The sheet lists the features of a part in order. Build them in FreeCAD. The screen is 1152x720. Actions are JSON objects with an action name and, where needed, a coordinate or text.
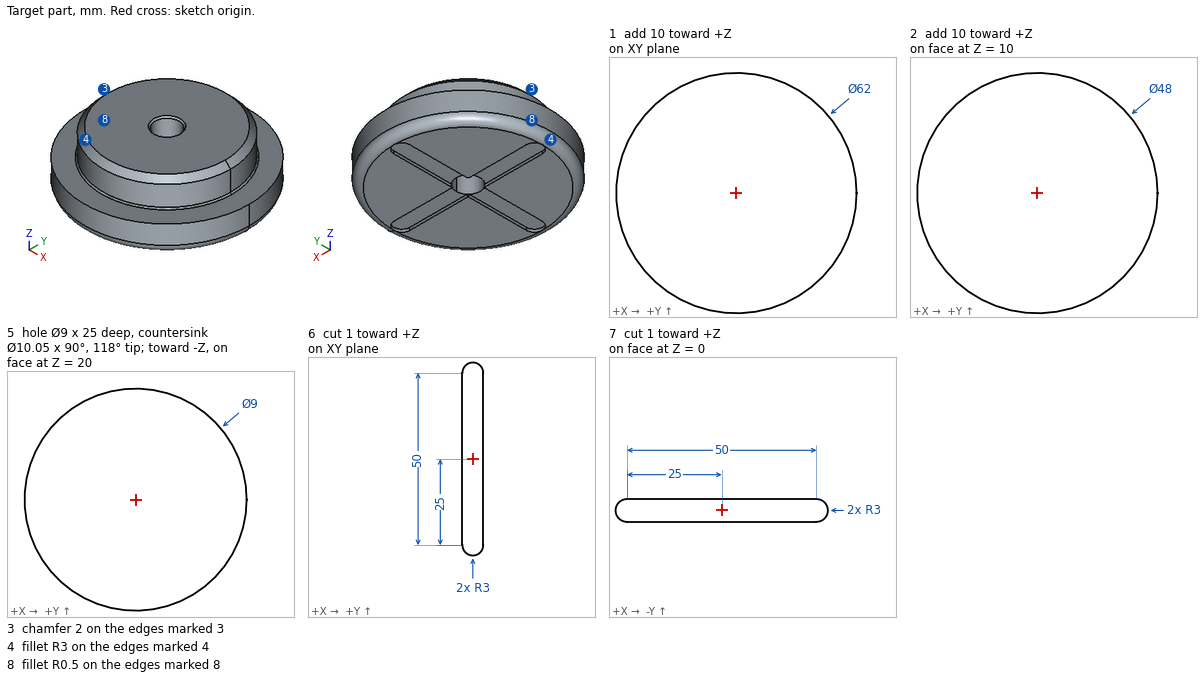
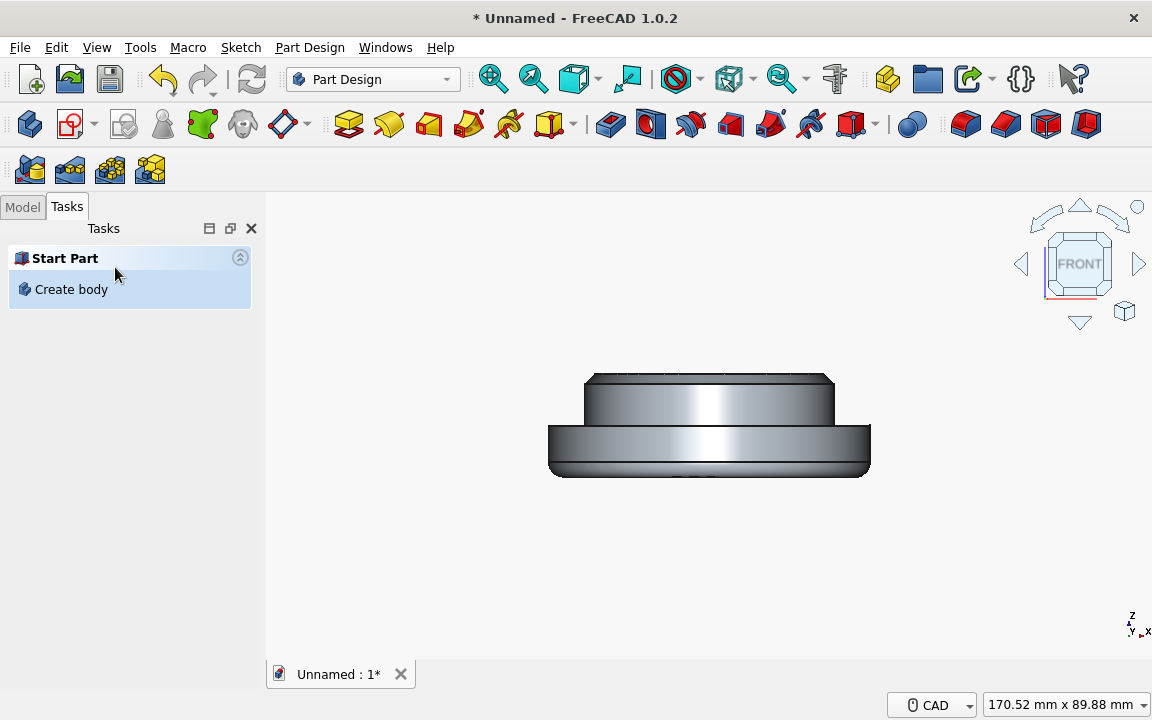
{"action": "left_click", "coordinate": [494, 80]}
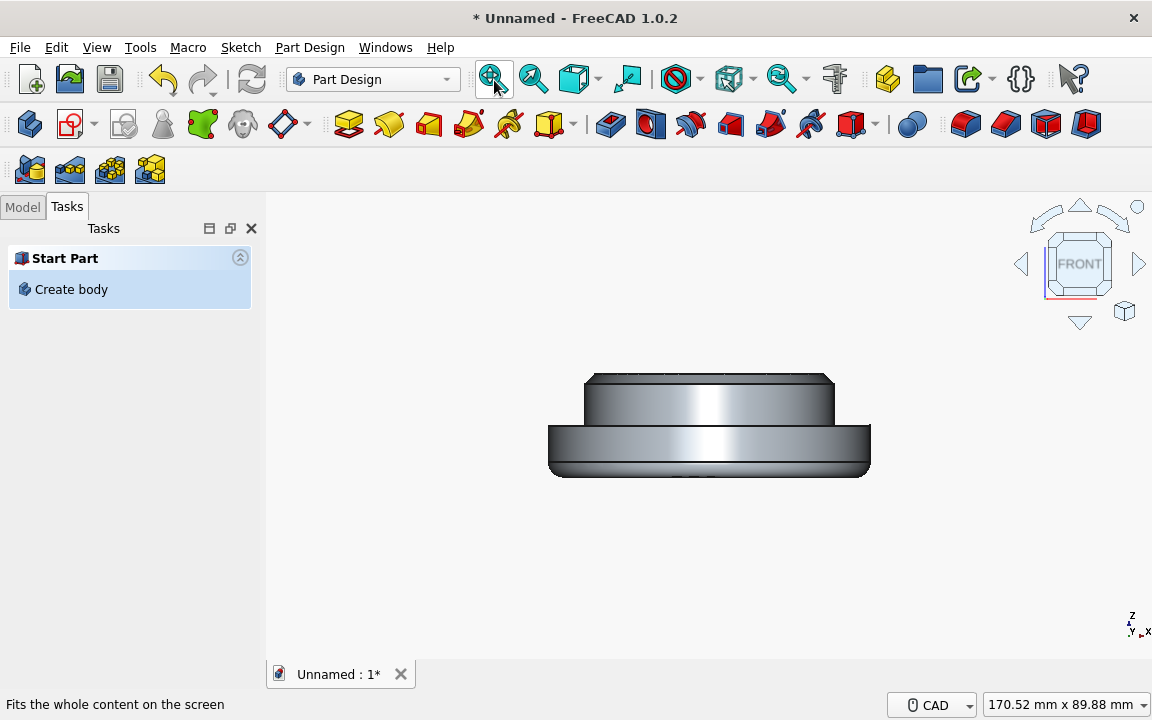
{"action": "key", "text": "3"}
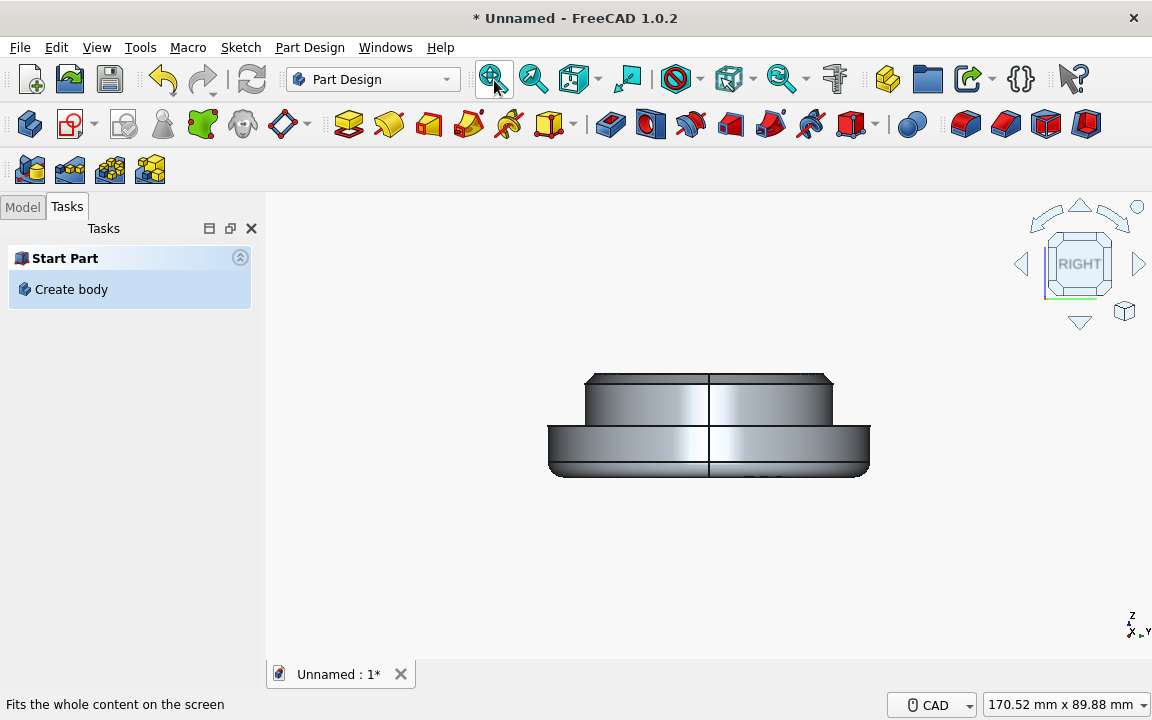
{"action": "left_click", "coordinate": [494, 80]}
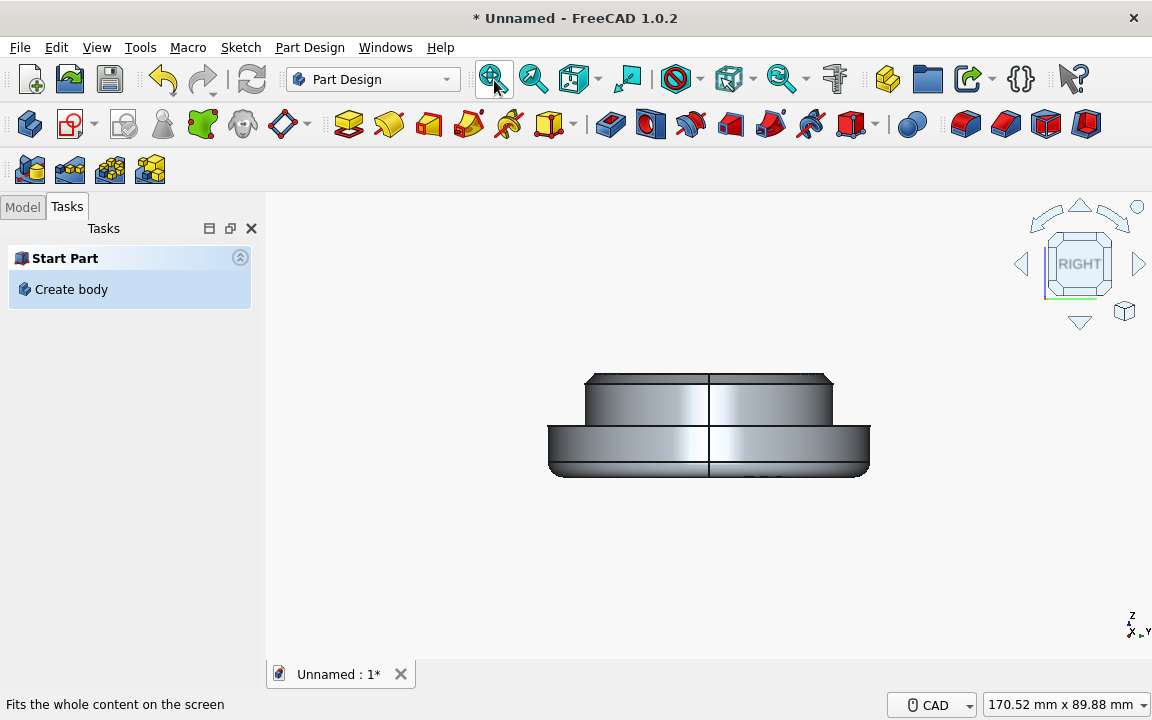
{"action": "key", "text": "5"}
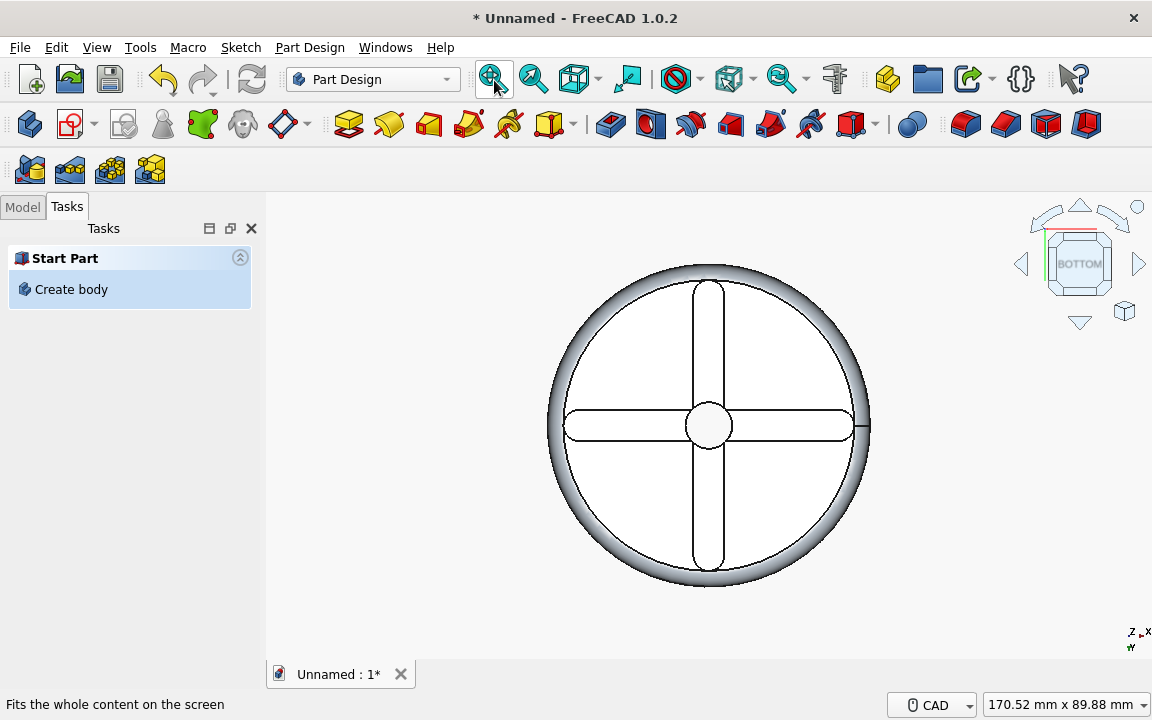
{"action": "key", "text": "4"}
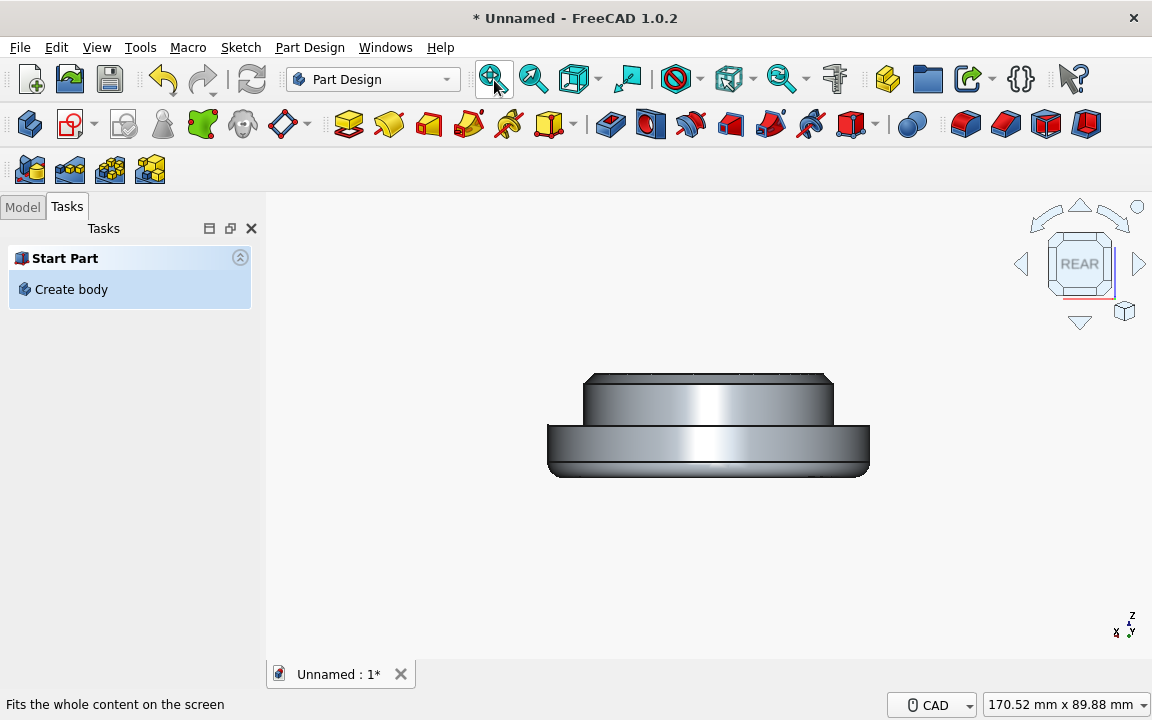
{"action": "left_click", "coordinate": [494, 80]}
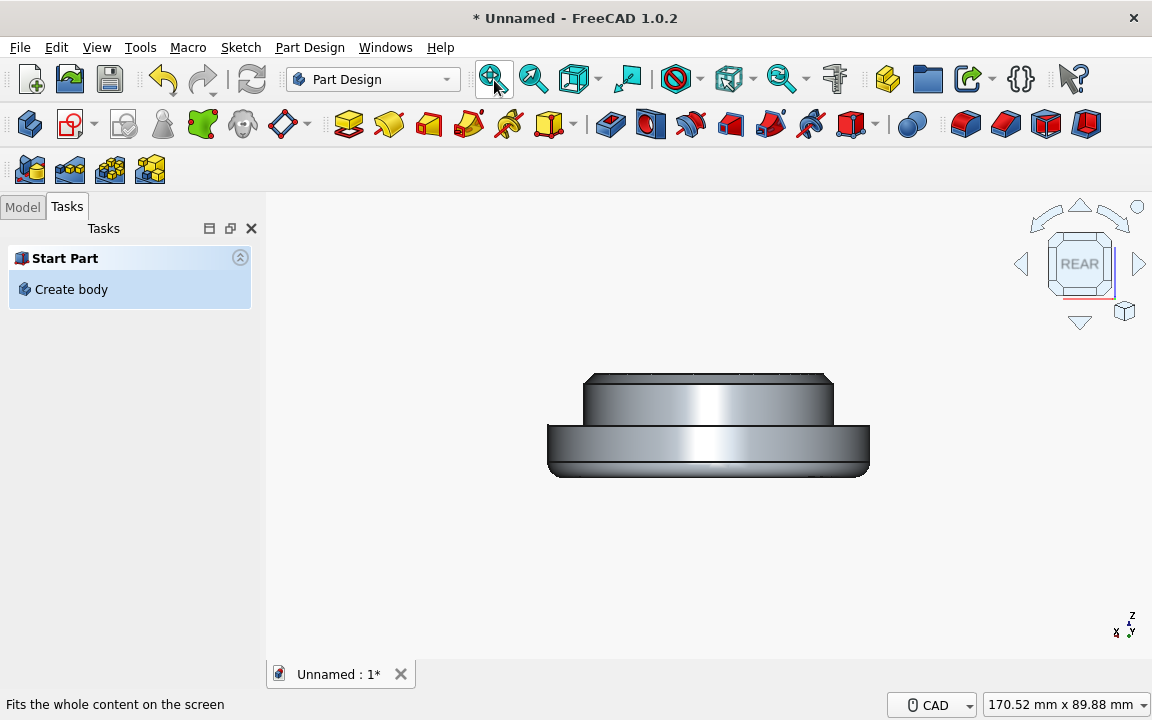
{"action": "key", "text": "6"}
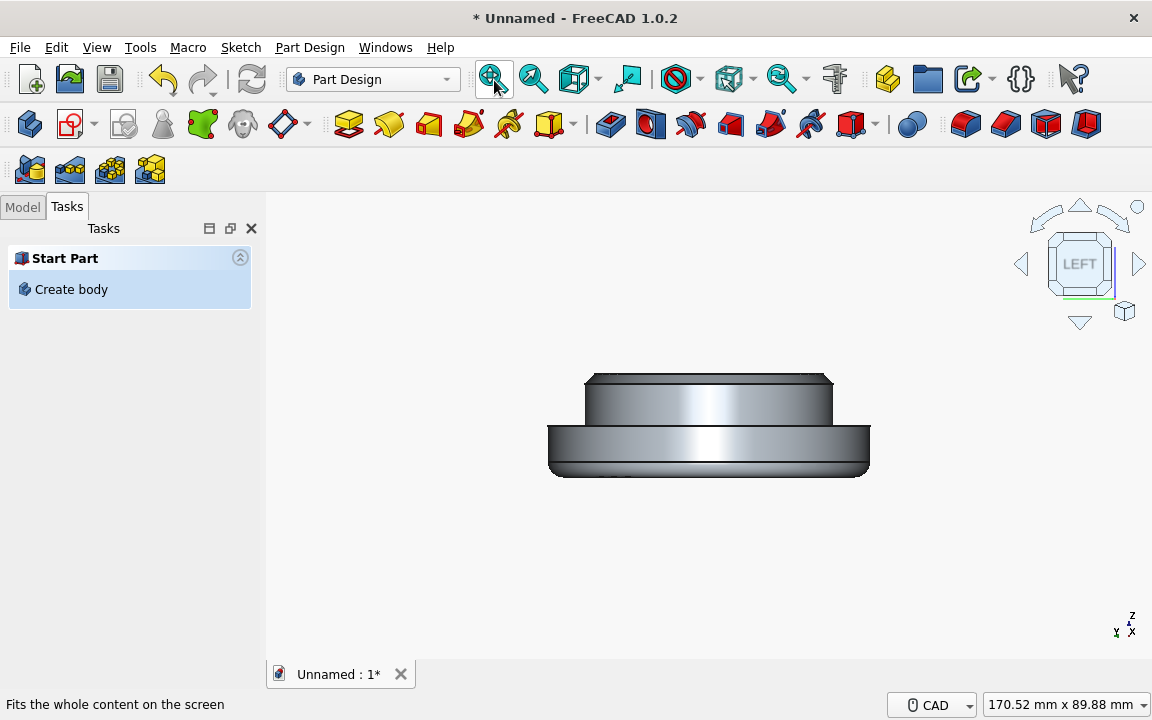
{"action": "left_click", "coordinate": [494, 80]}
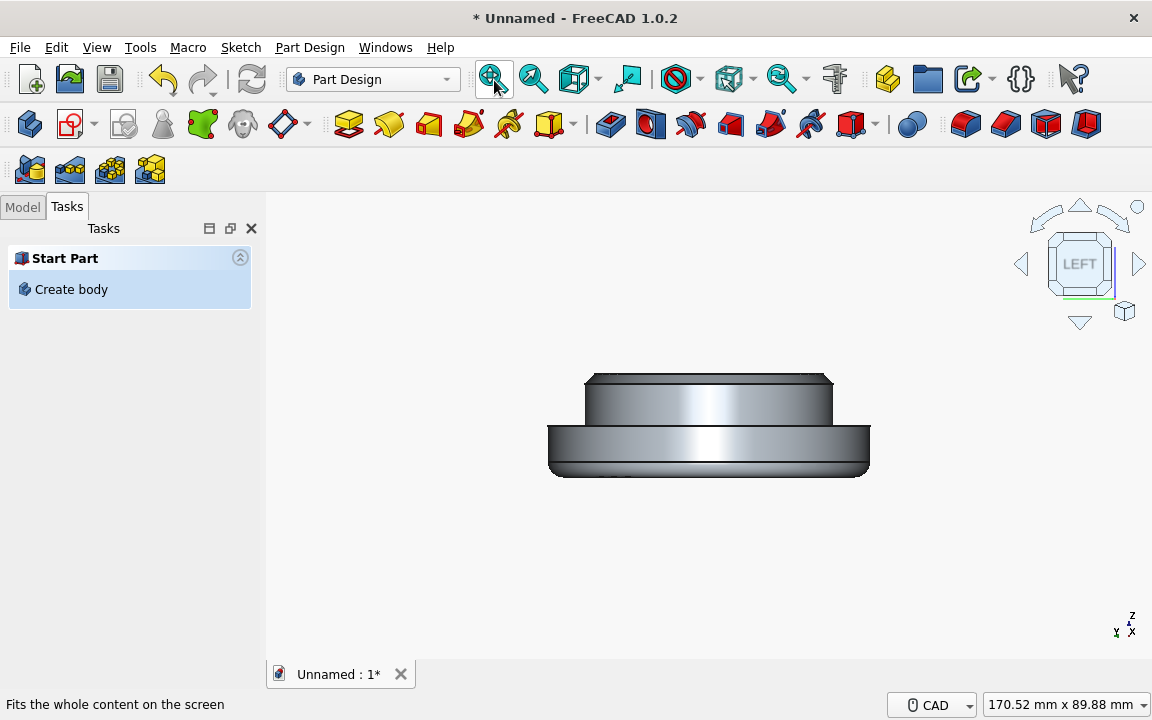
{"action": "key", "text": "v 3"}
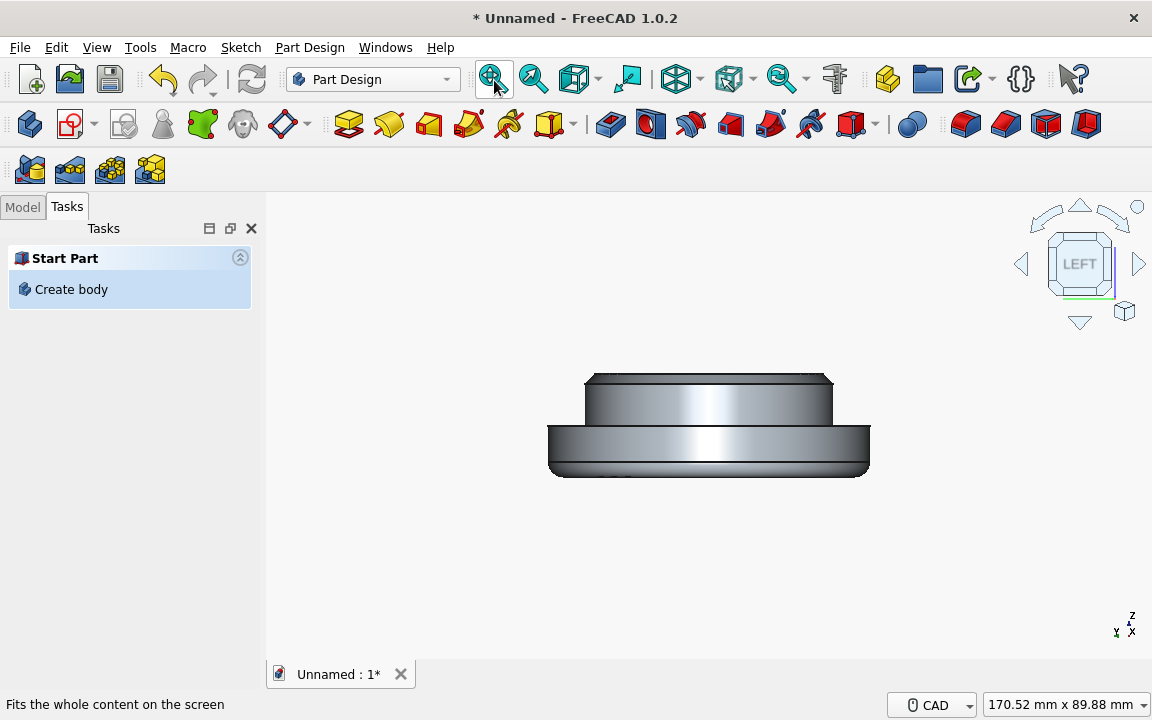
{"action": "key", "text": "0"}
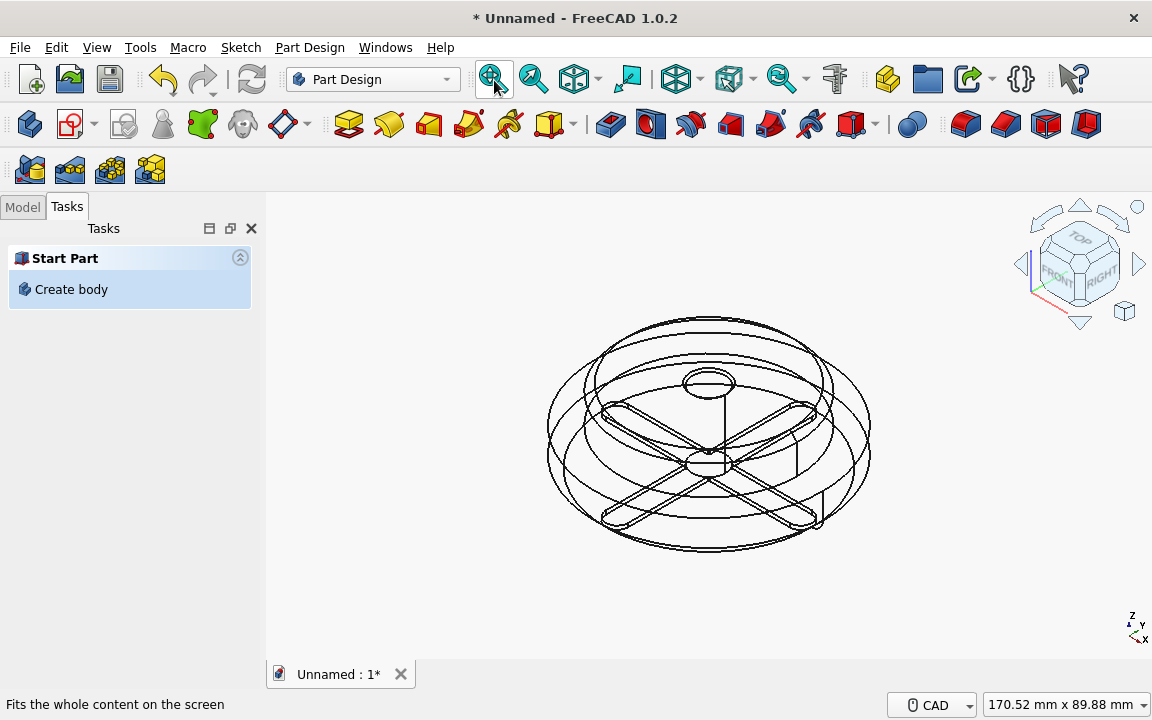
{"action": "left_click", "coordinate": [621, 374]}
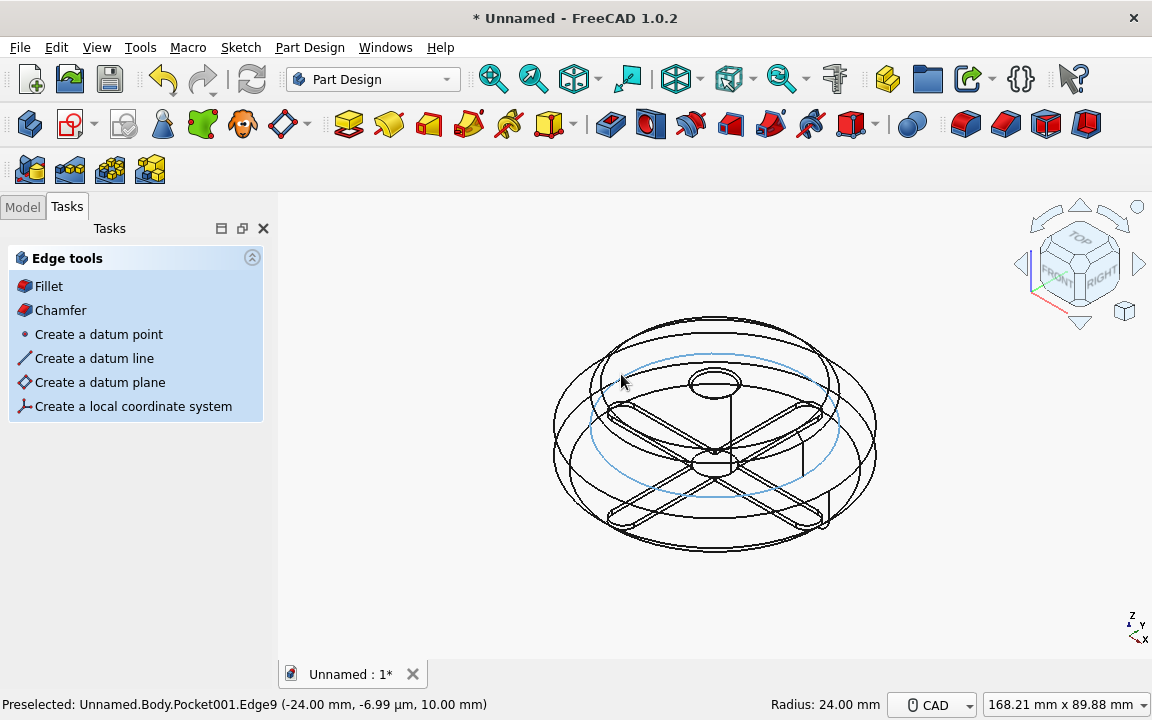
{"action": "key", "text": "v 1"}